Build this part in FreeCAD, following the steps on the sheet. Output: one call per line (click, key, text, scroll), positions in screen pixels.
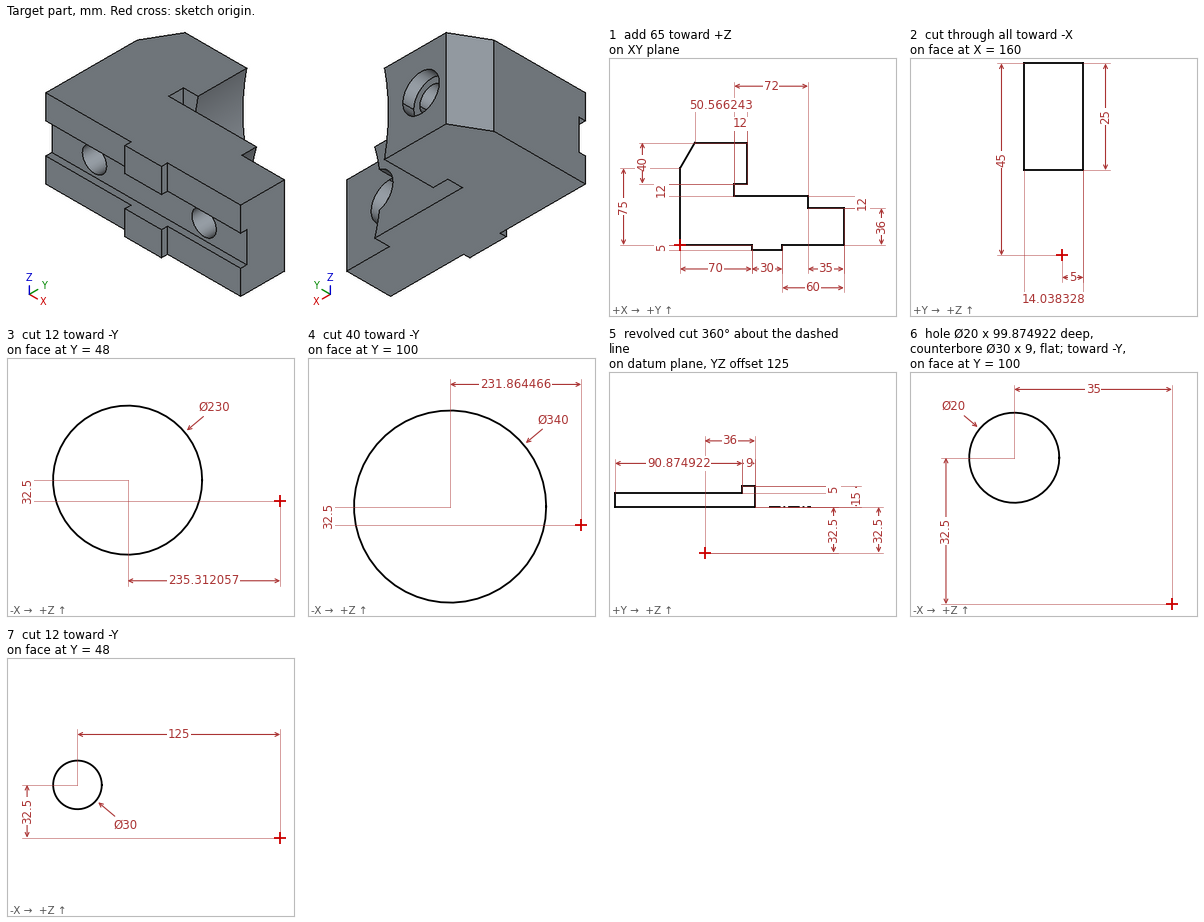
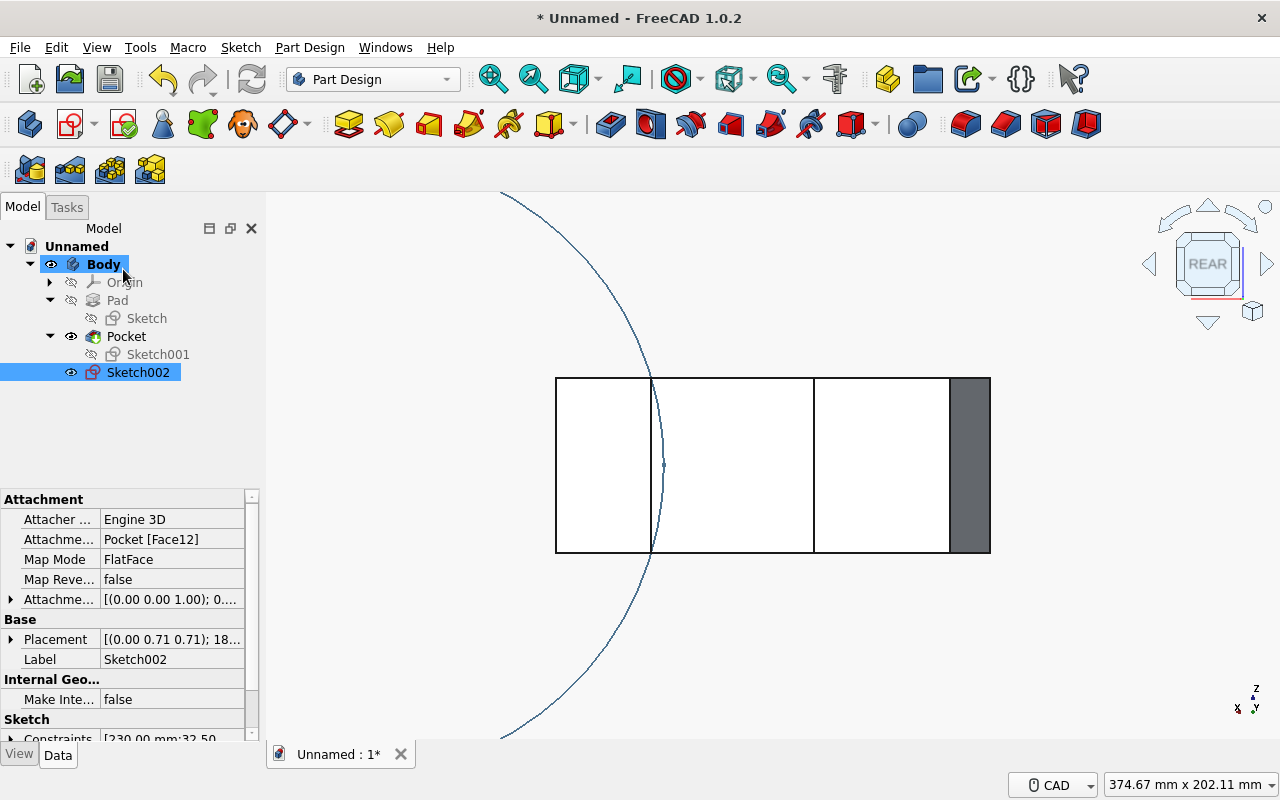
click(612, 124)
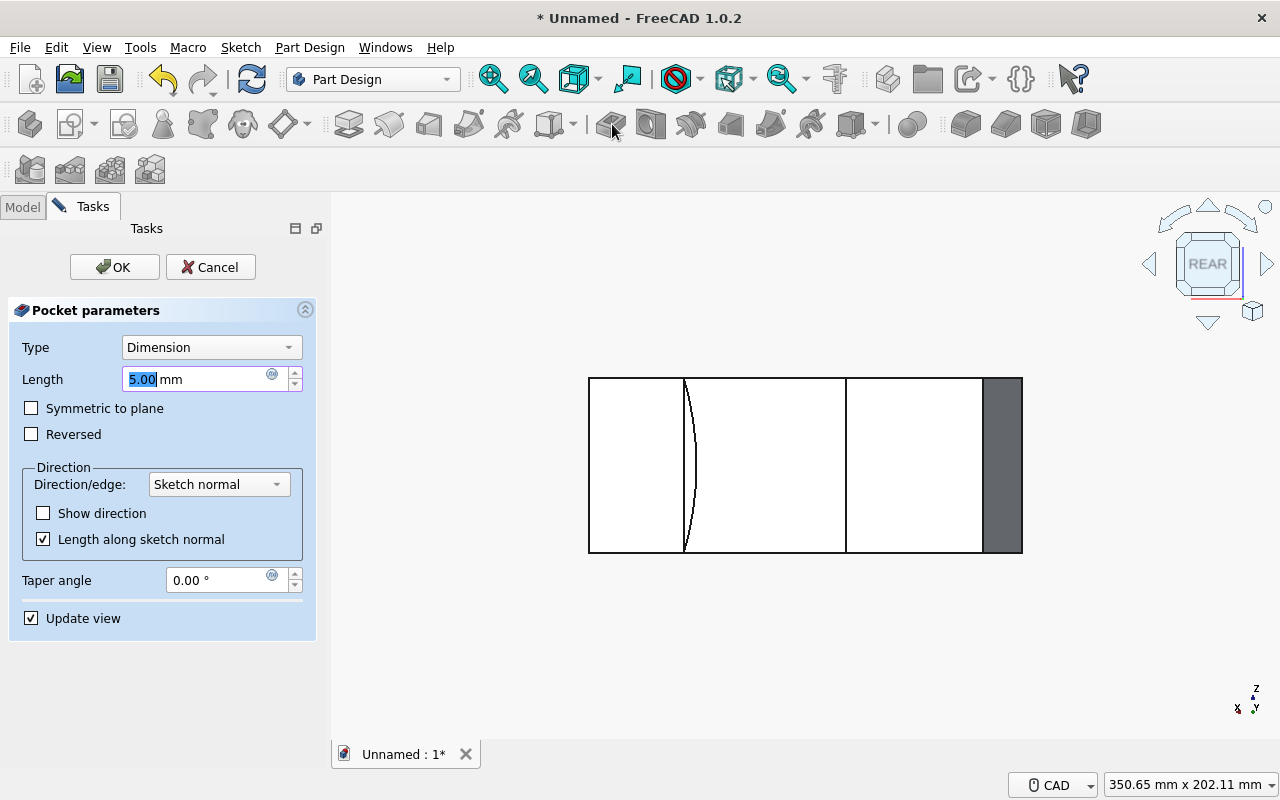
text(12)
key(Tab)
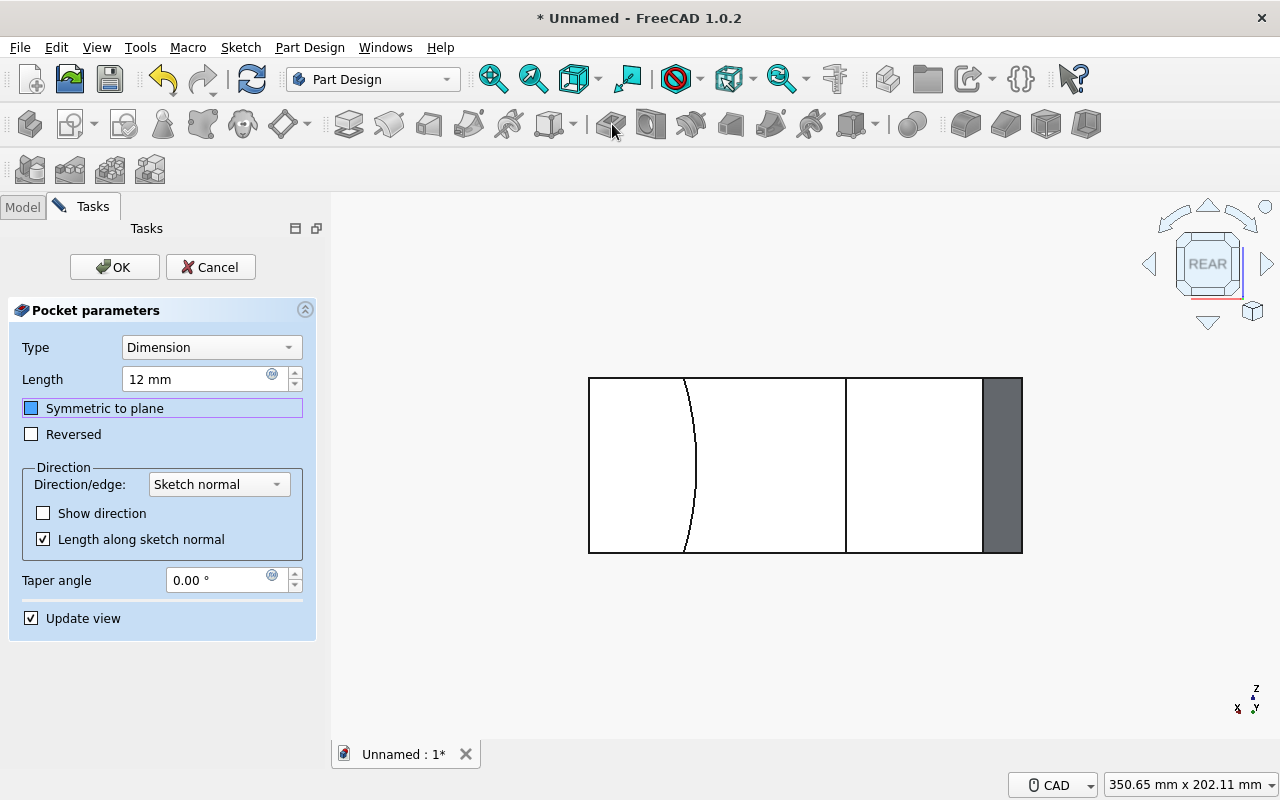
click(115, 267)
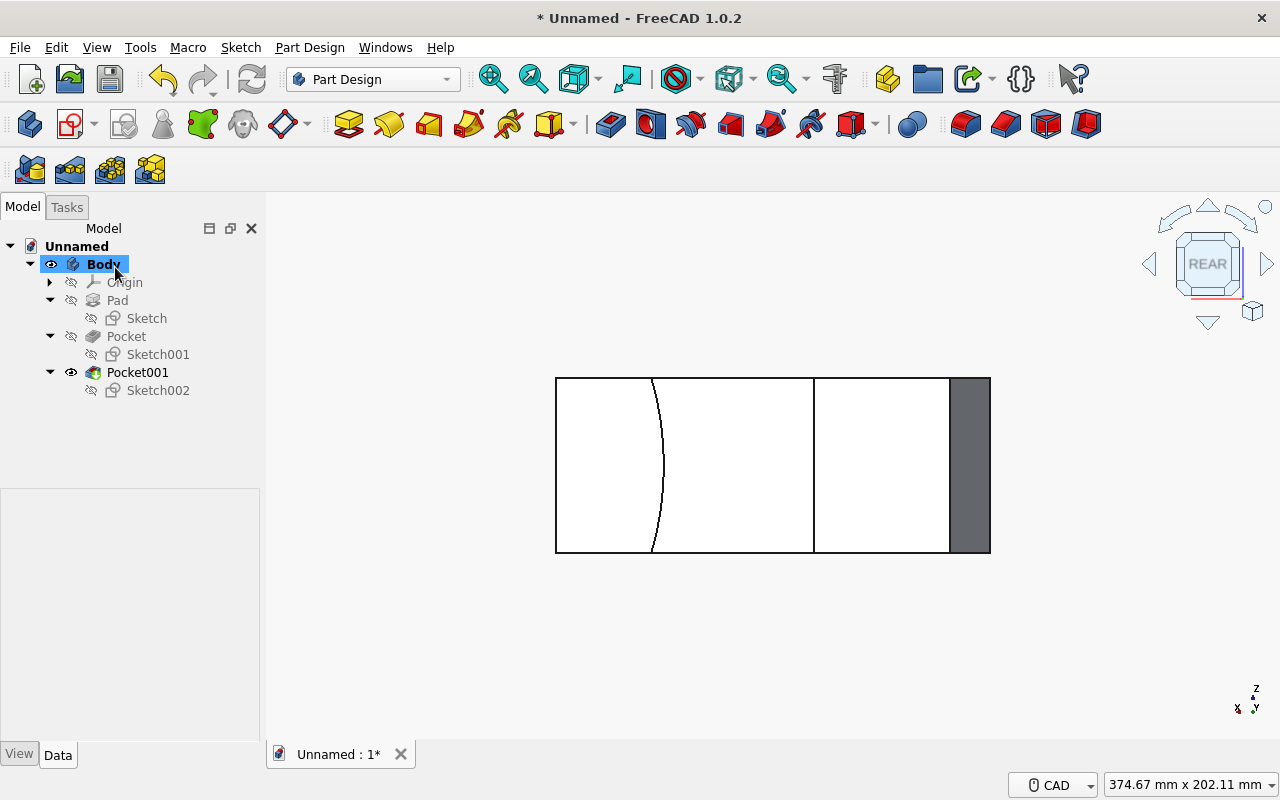
click(494, 80)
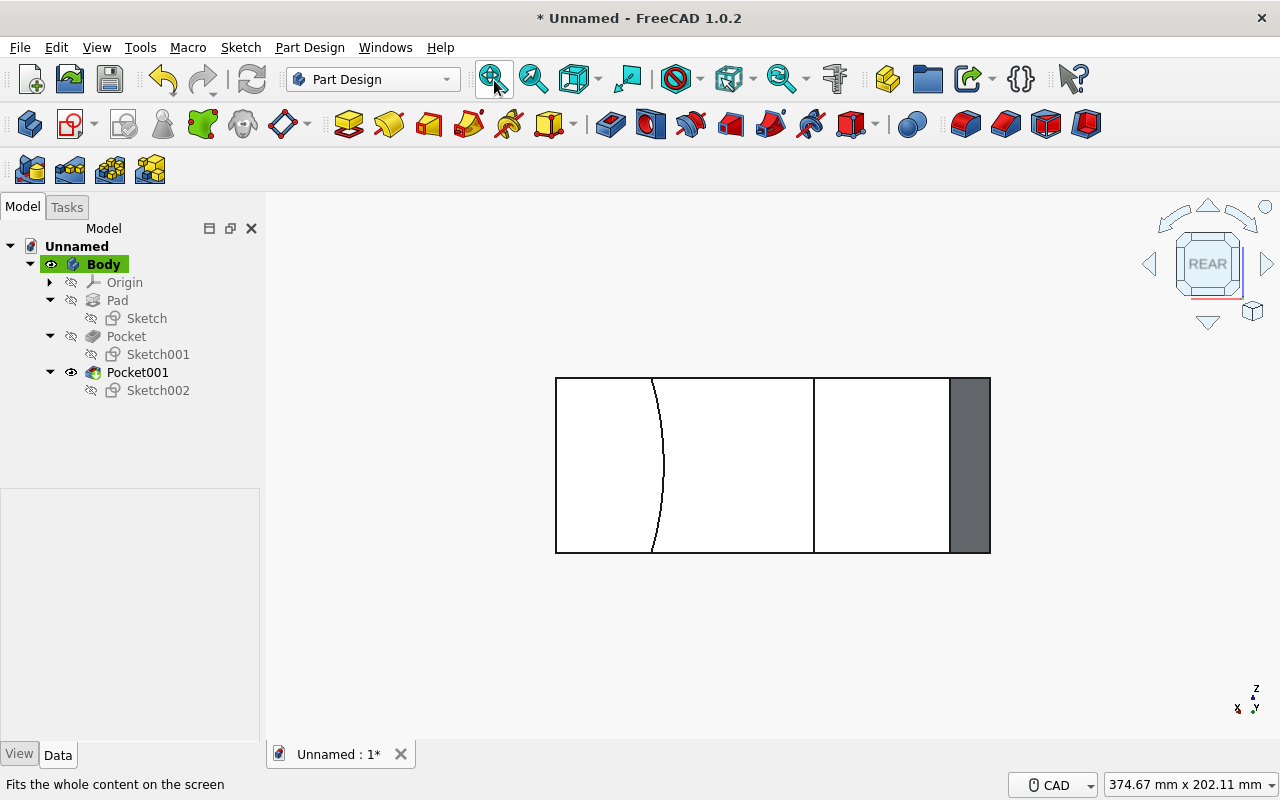
click(882, 464)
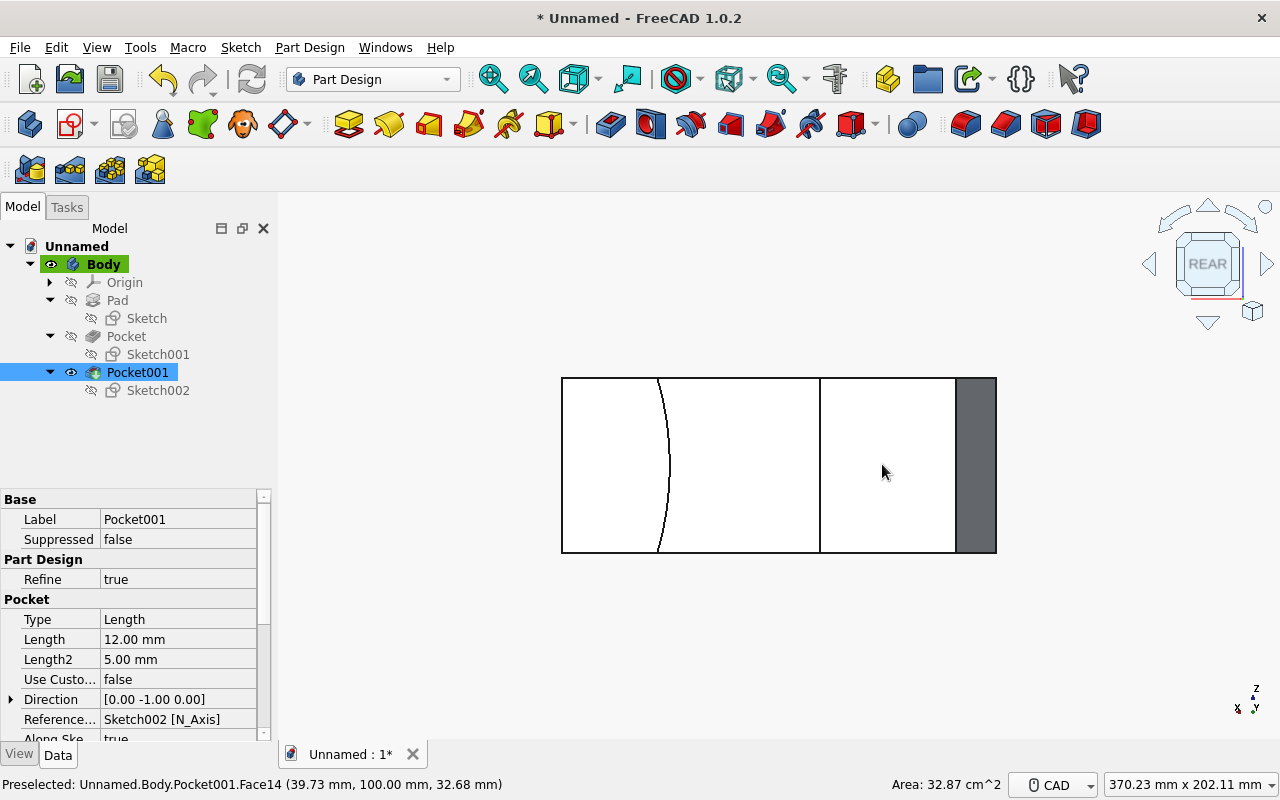
click(70, 124)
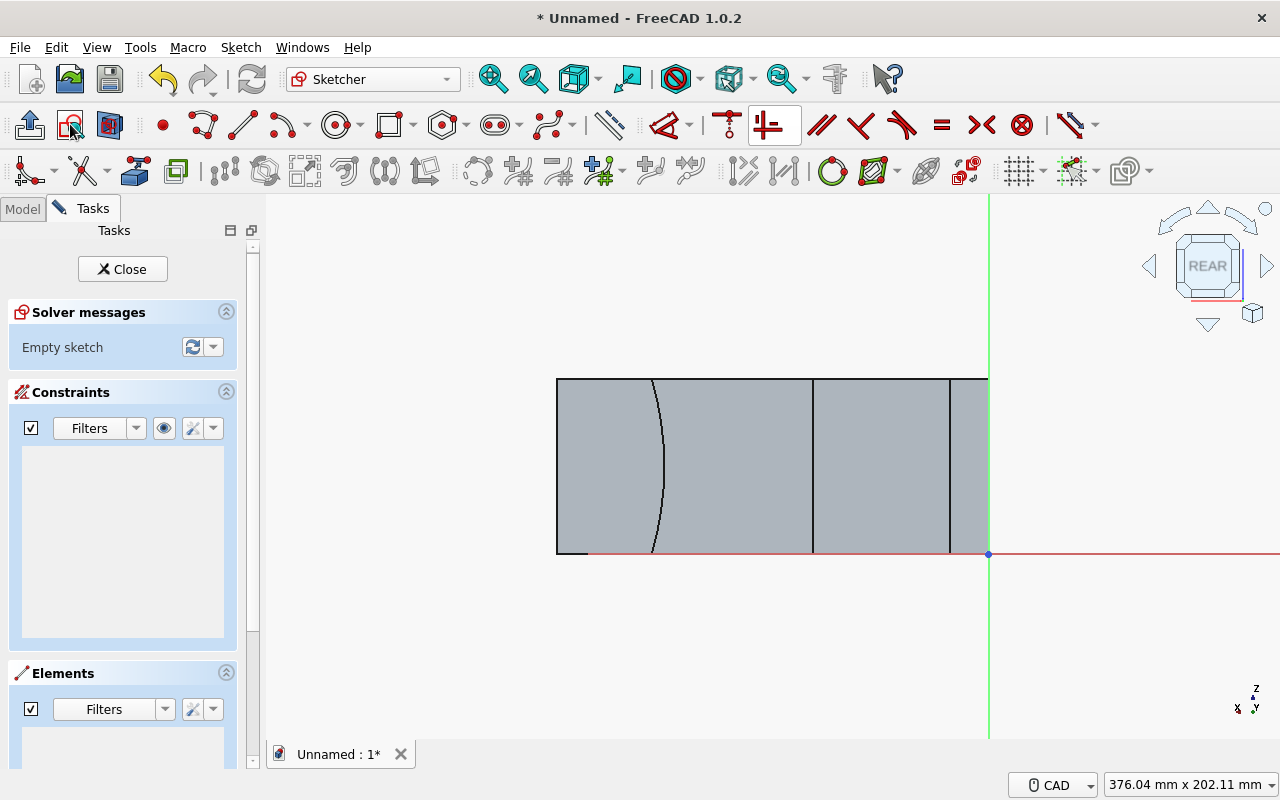
scroll(854, 466, down, 5)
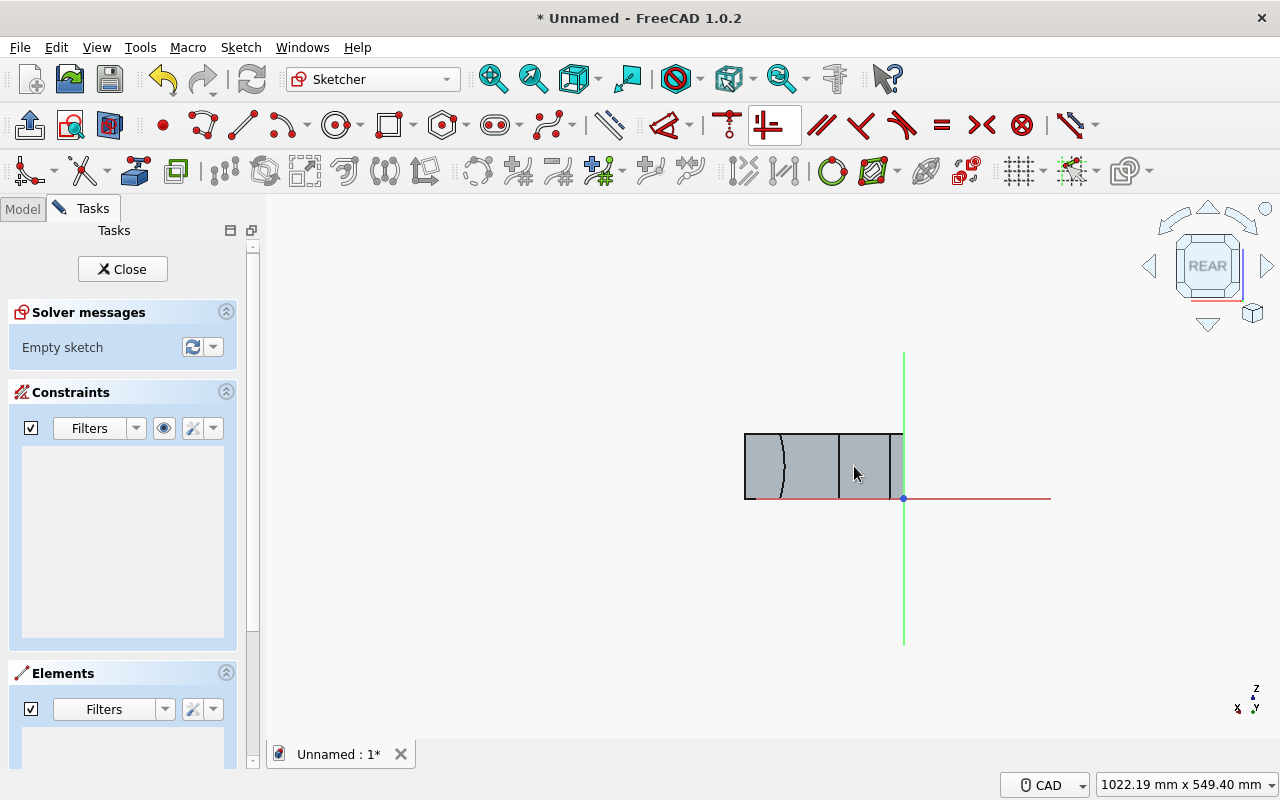
key(g)
key(c)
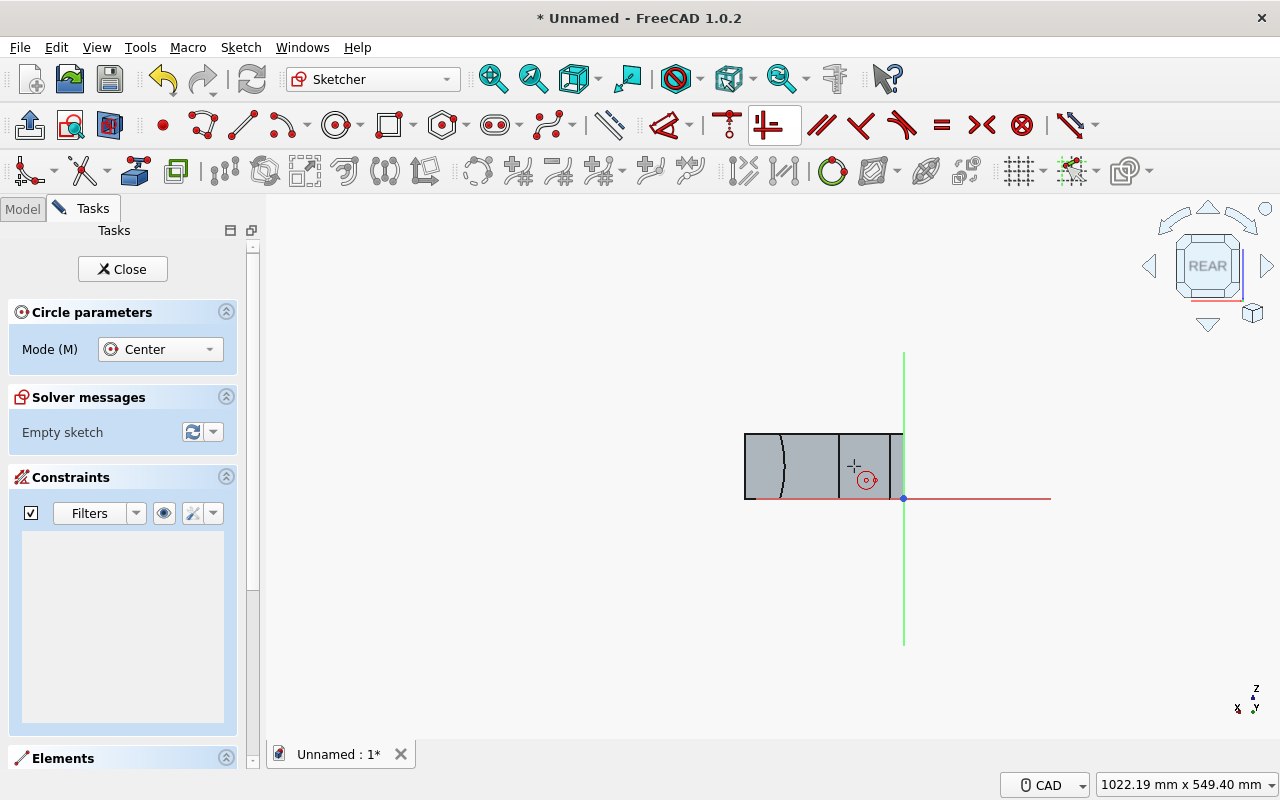
click(674, 466)
move(793, 347)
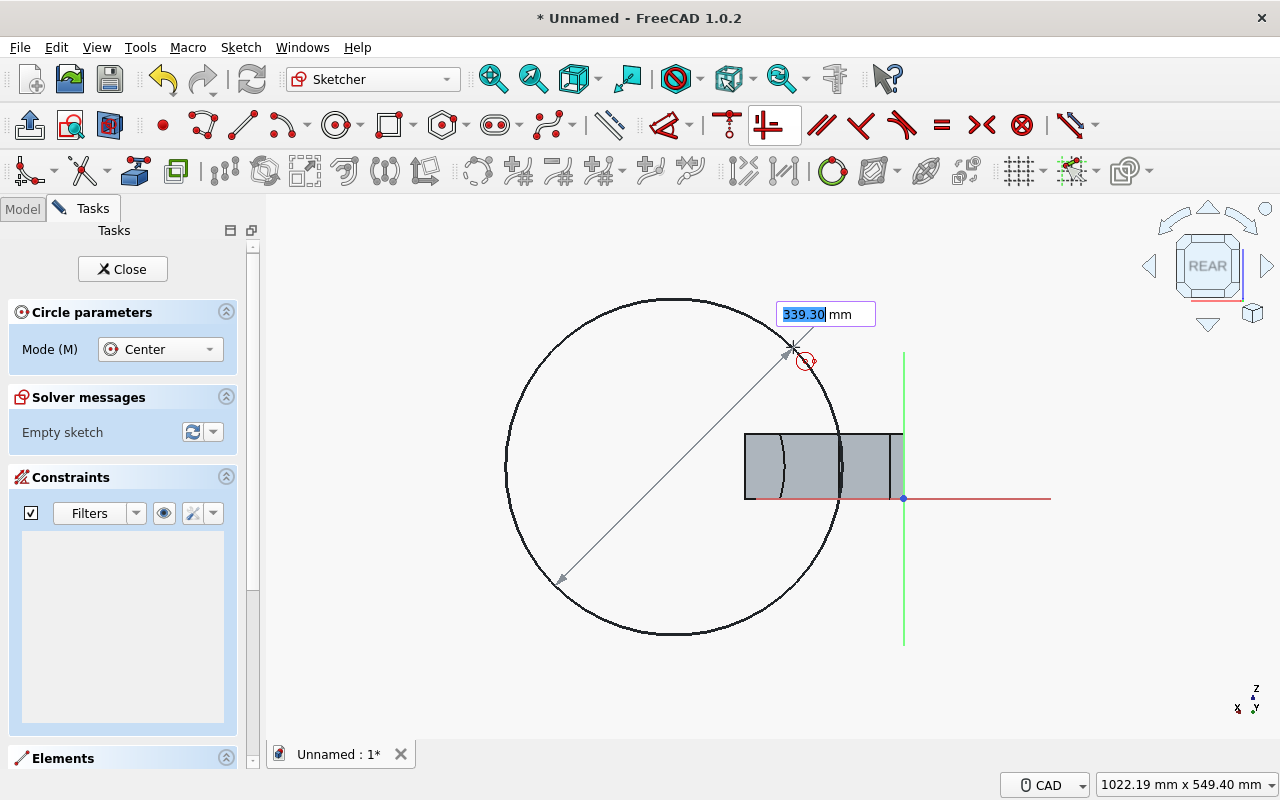
text(340)
key(Return)
key(Escape)